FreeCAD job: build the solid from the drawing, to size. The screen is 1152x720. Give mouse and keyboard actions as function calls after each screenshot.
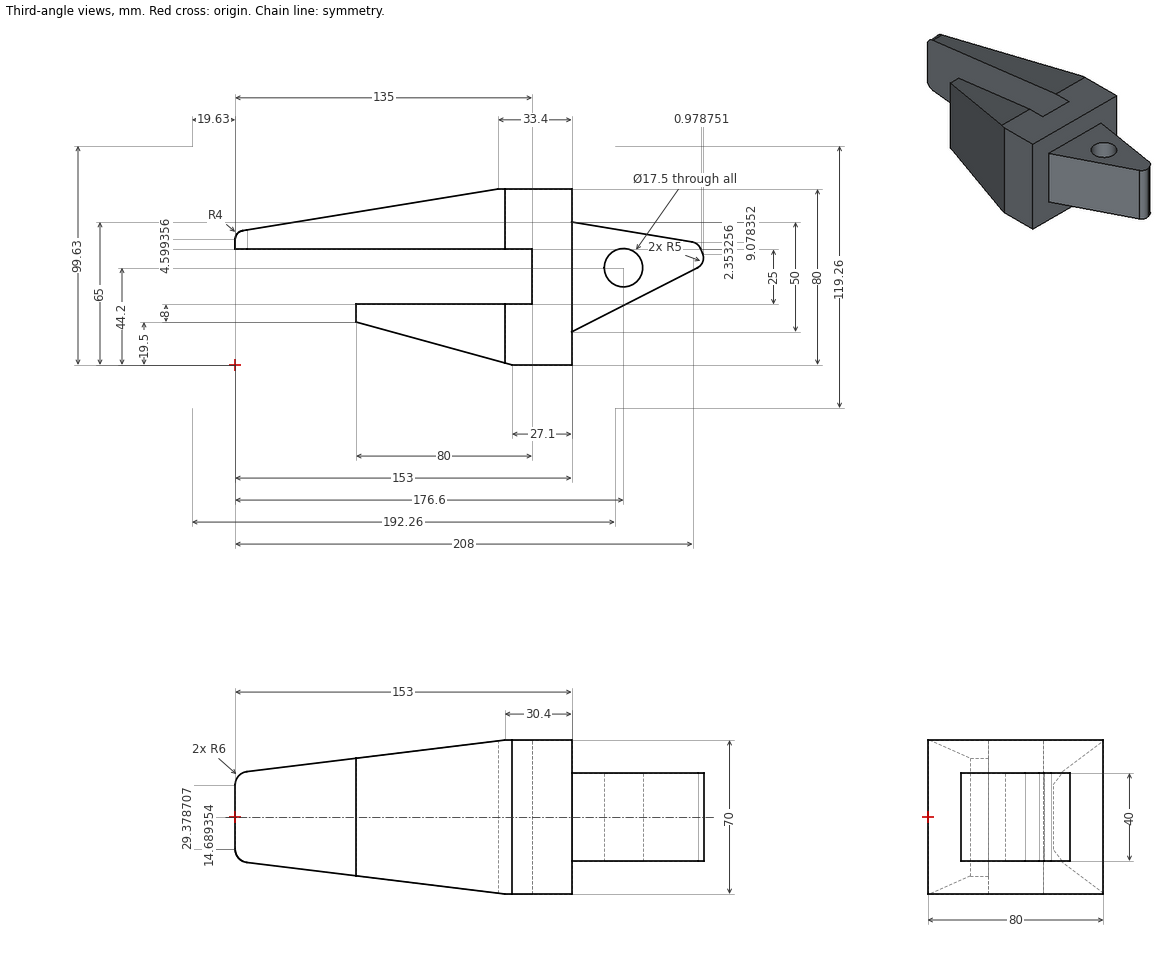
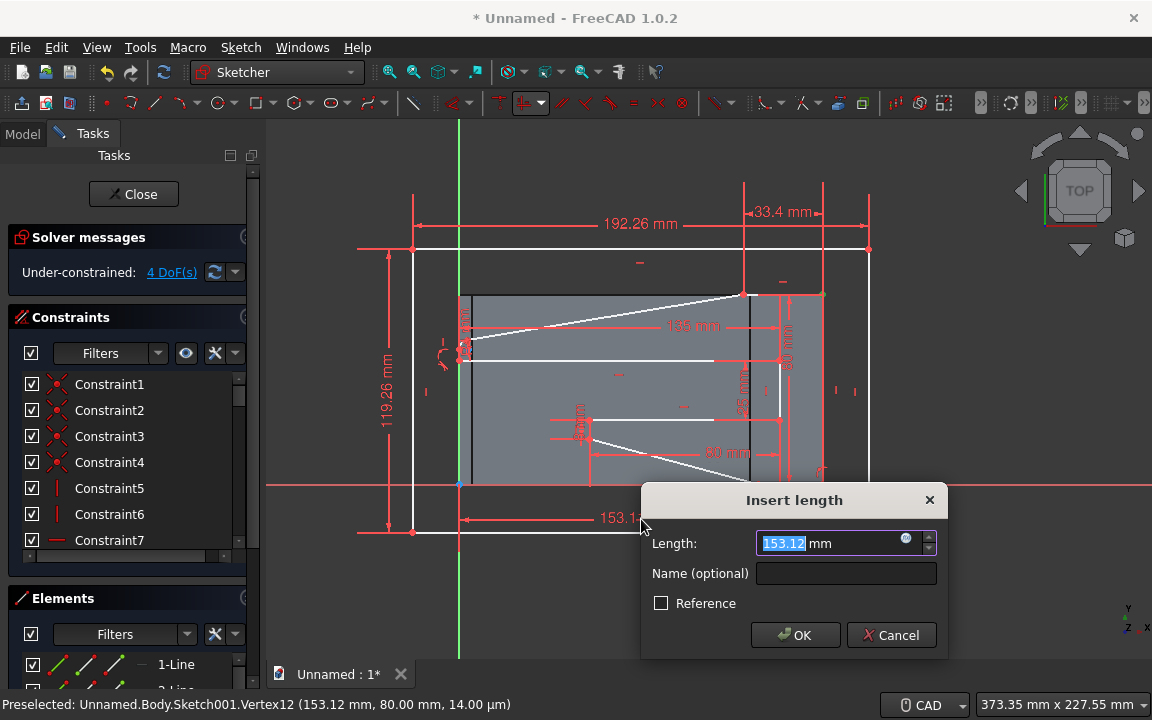
text(153)
key(Return)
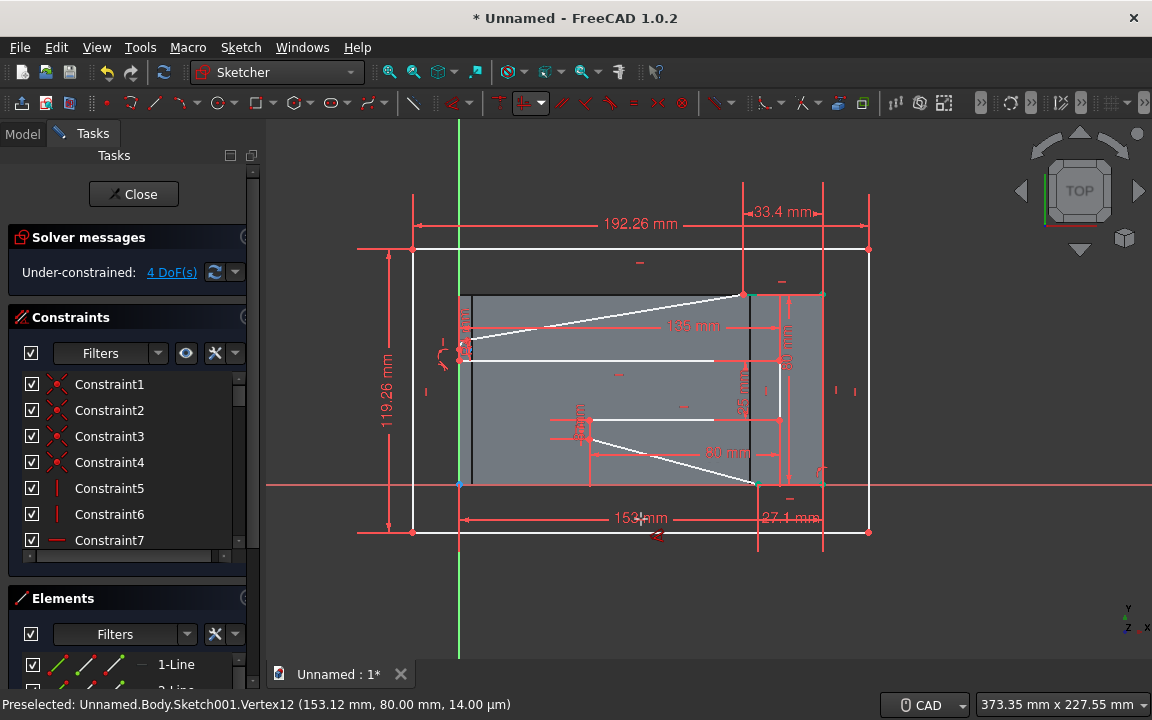
click(590, 439)
click(624, 462)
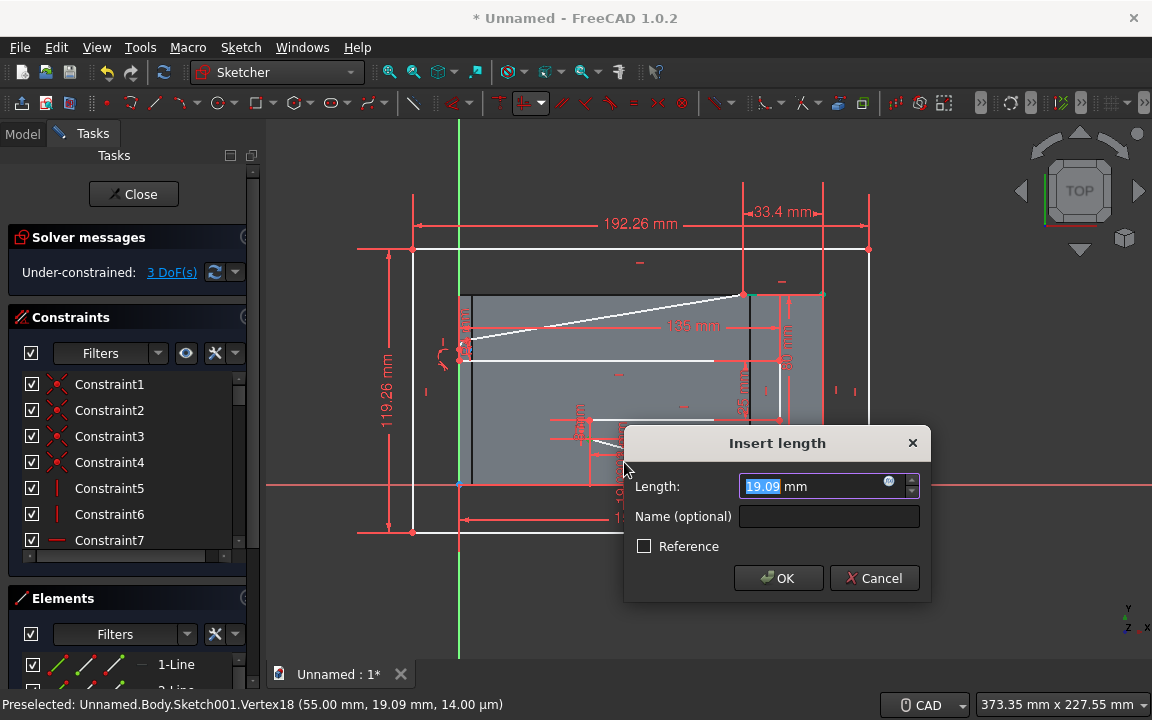
text(19.5)
key(Return)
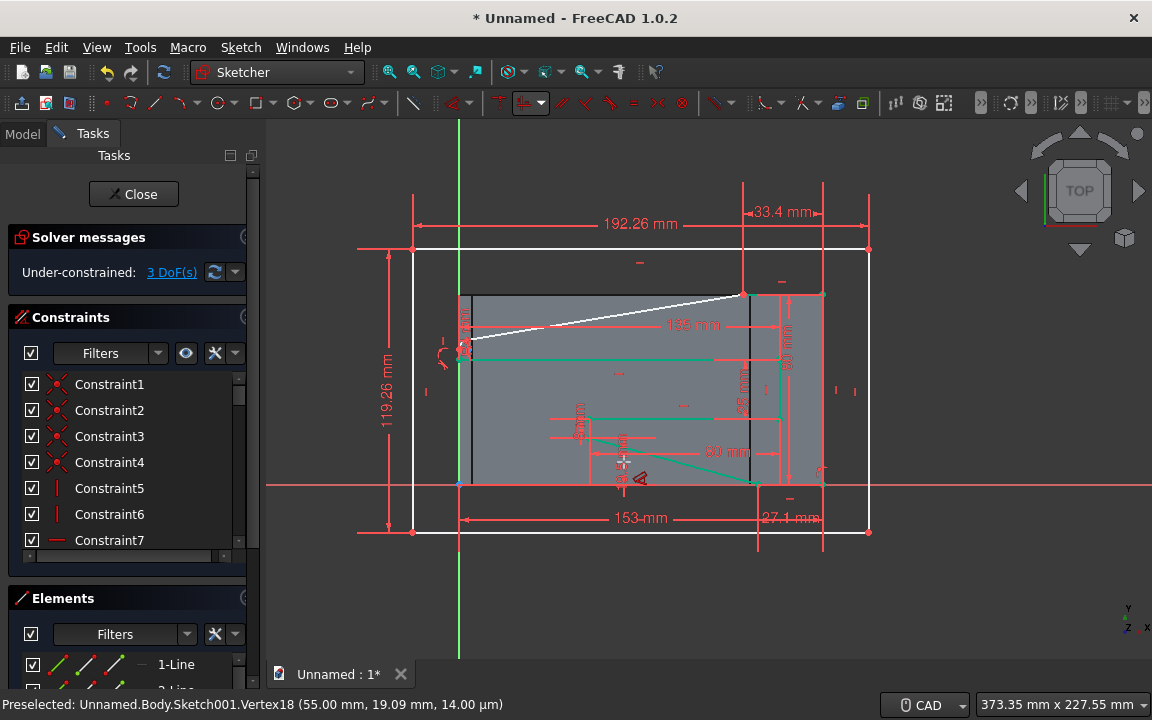
click(413, 249)
click(436, 215)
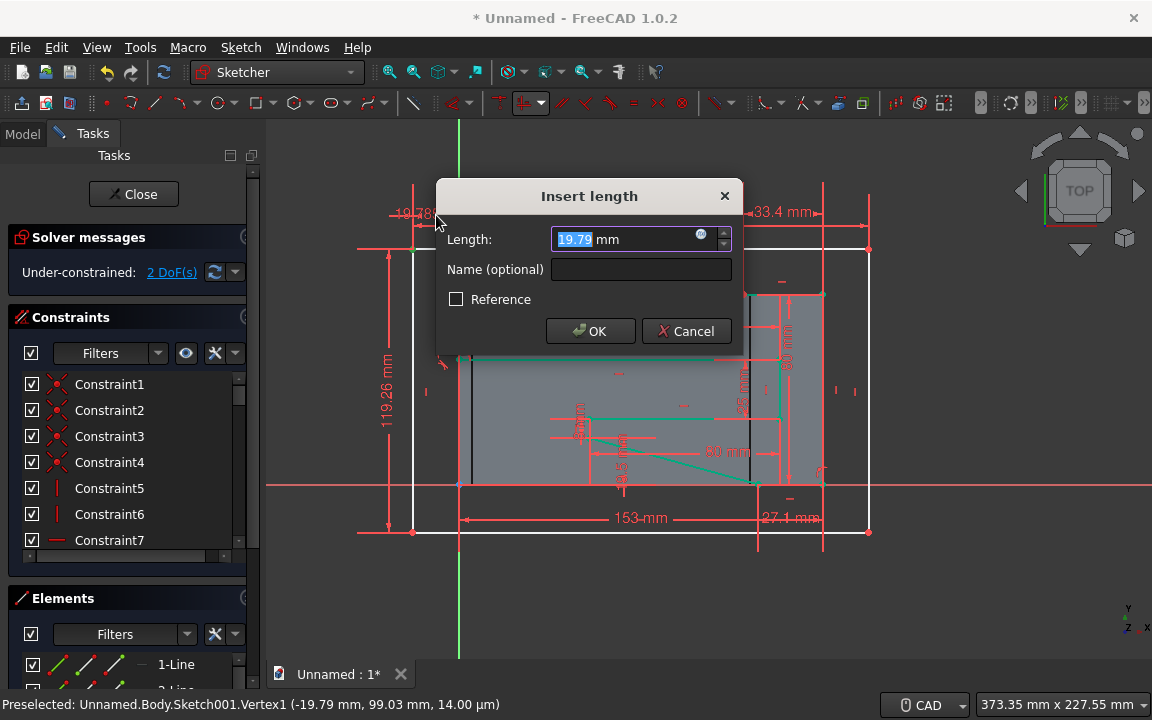
text(19.63)
key(Return)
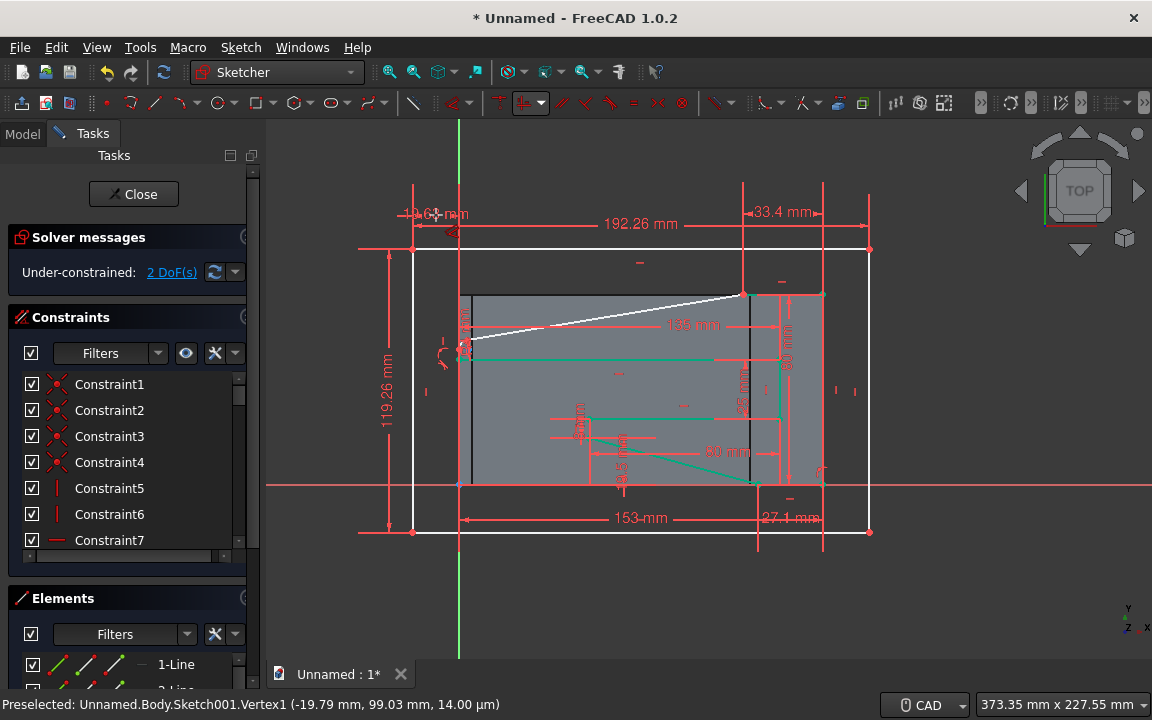
click(413, 249)
click(379, 367)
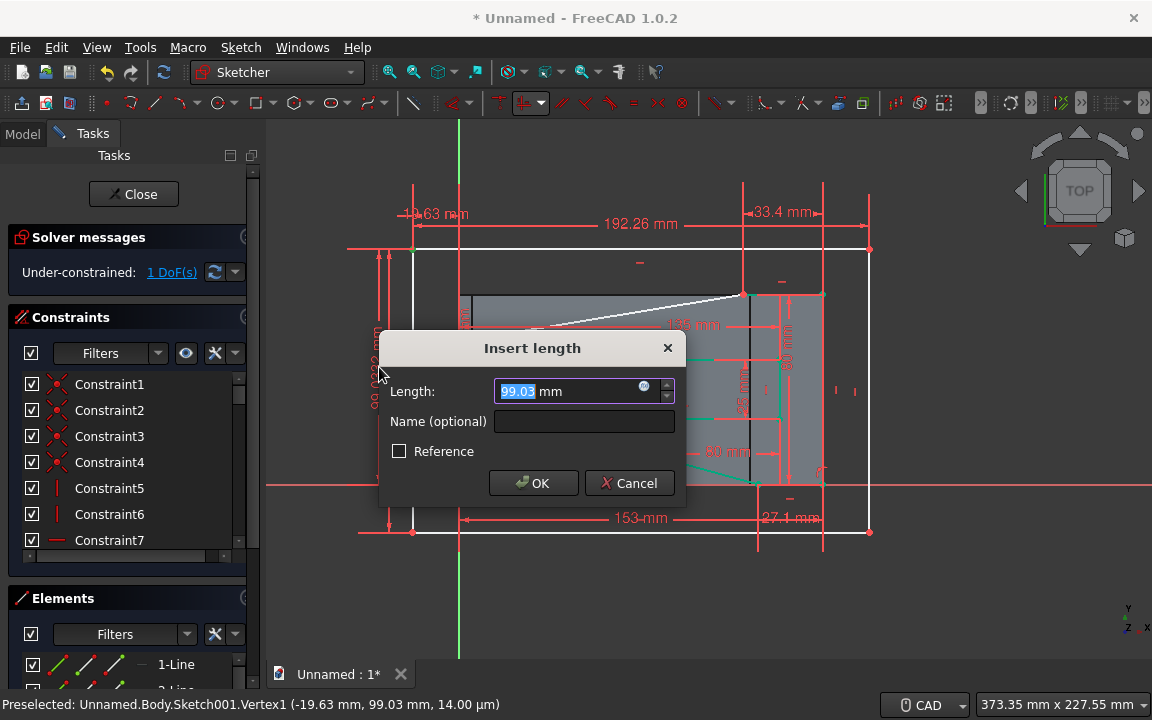
text(99.63)
key(Return)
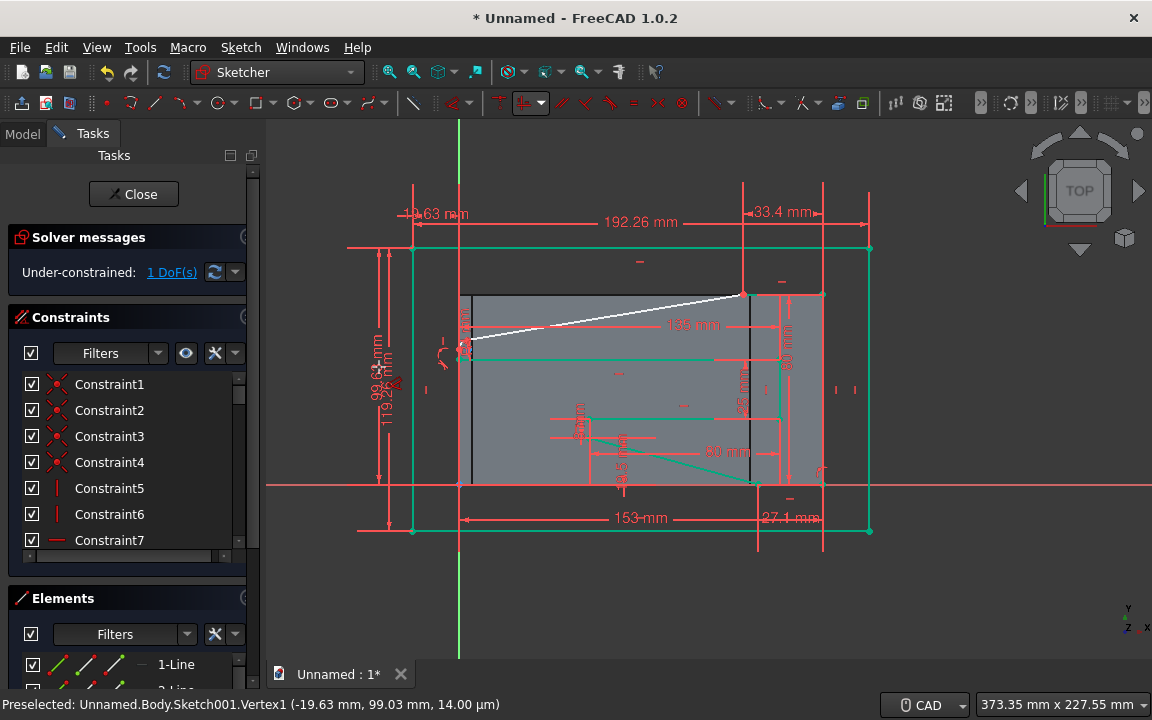
scroll(459, 355, up, 7)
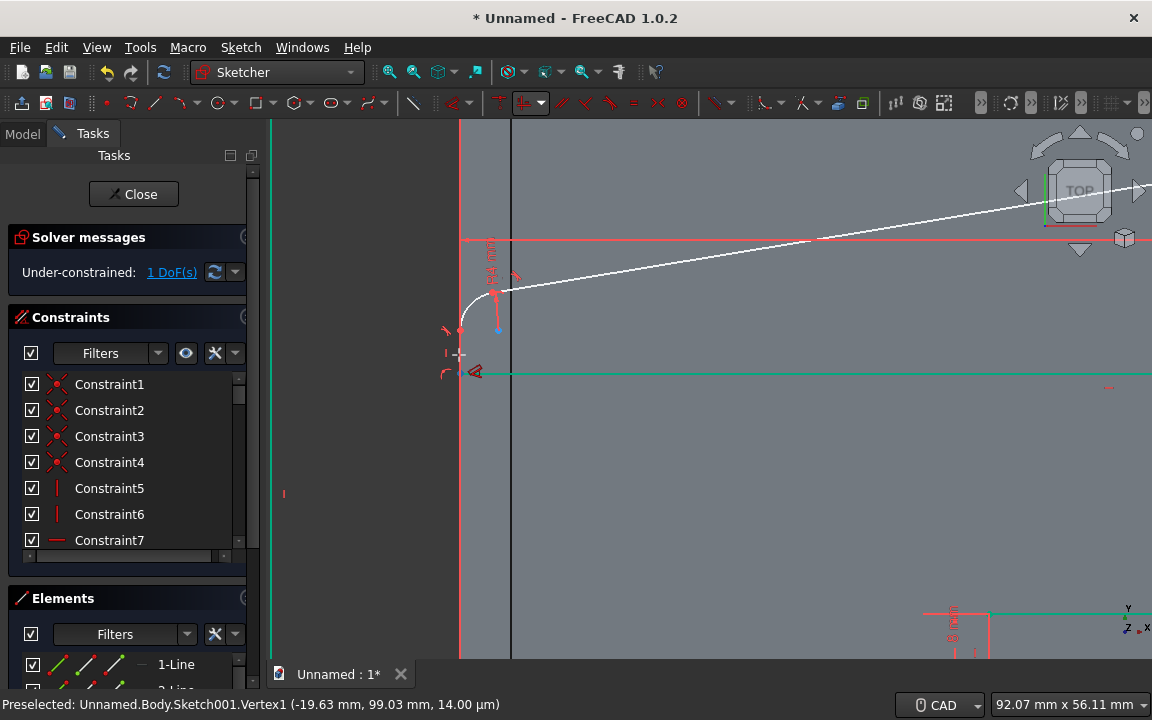
click(460, 352)
click(426, 352)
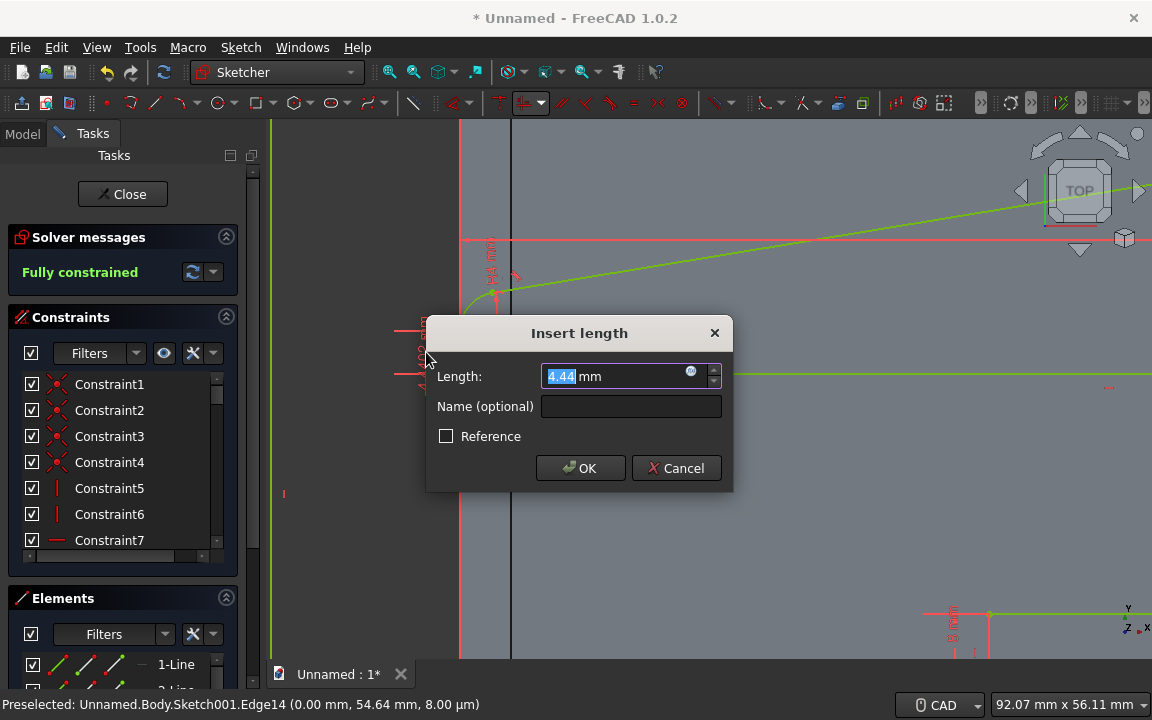
text(4.599356)
key(Return)
key(Escape)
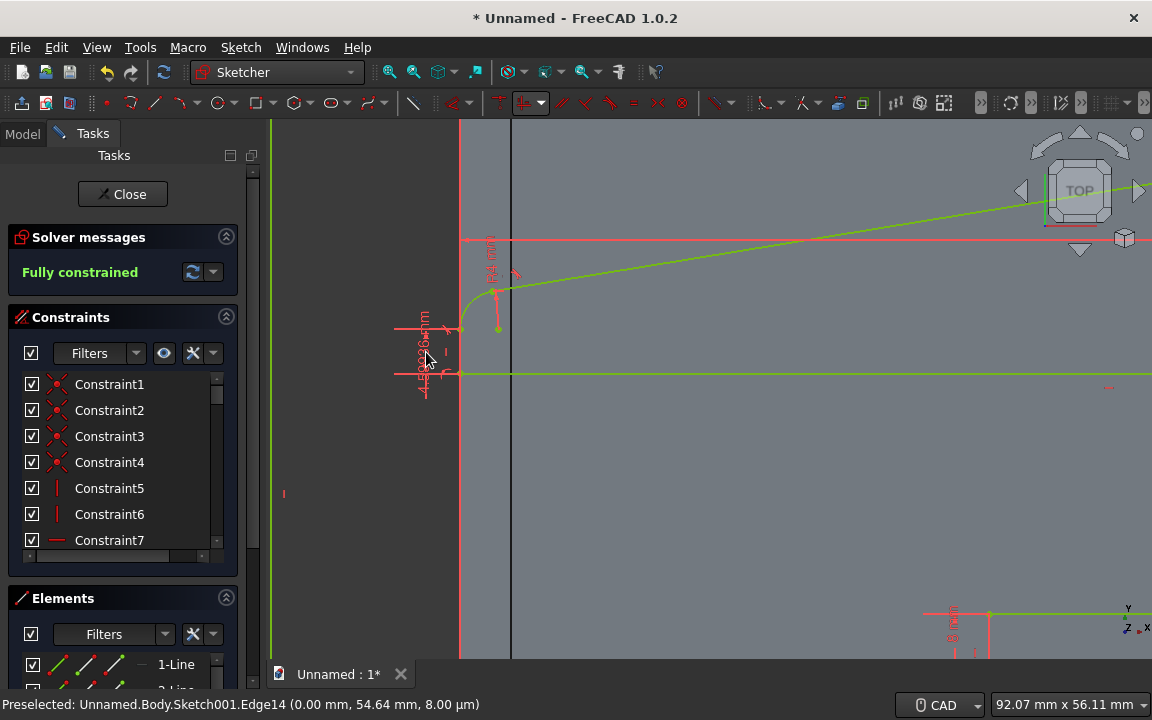
click(123, 194)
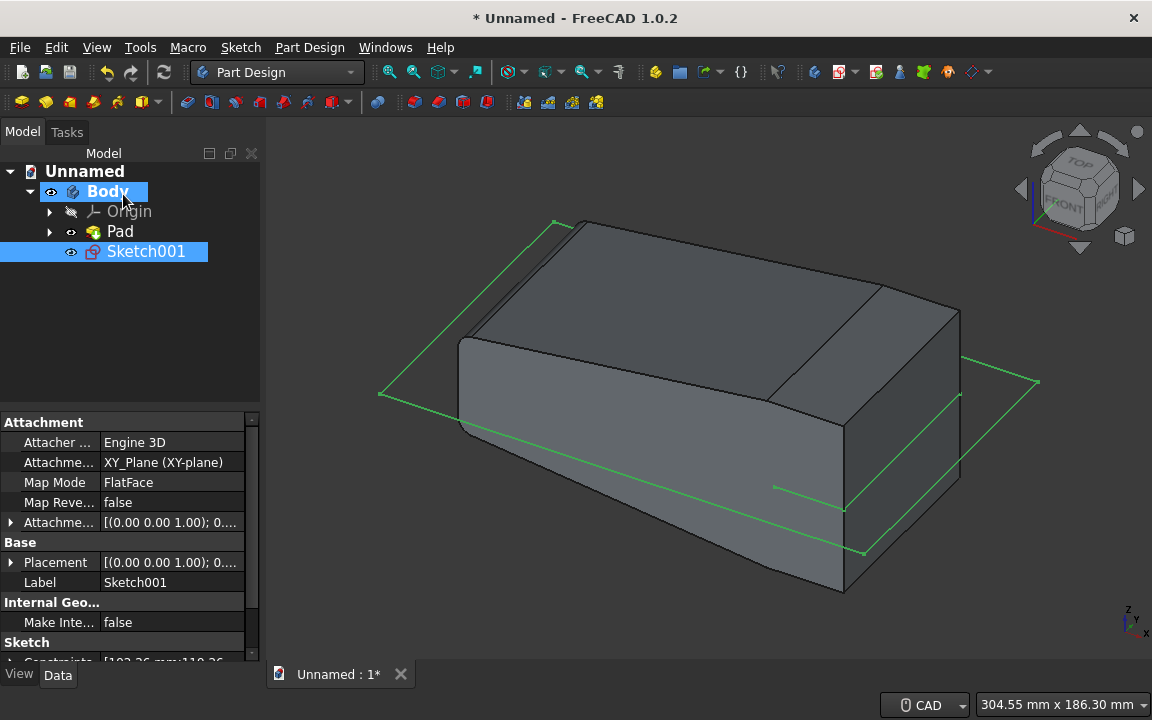
click(188, 102)